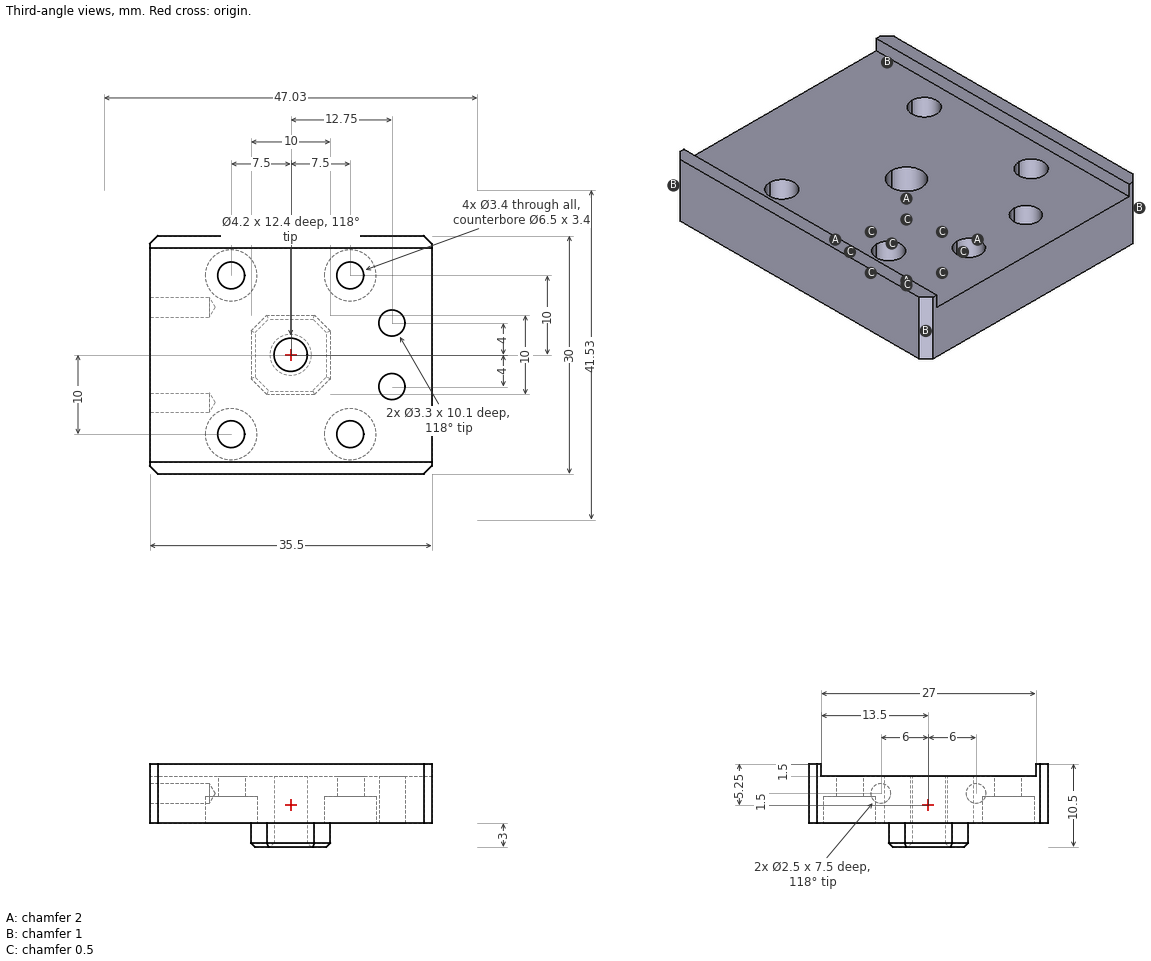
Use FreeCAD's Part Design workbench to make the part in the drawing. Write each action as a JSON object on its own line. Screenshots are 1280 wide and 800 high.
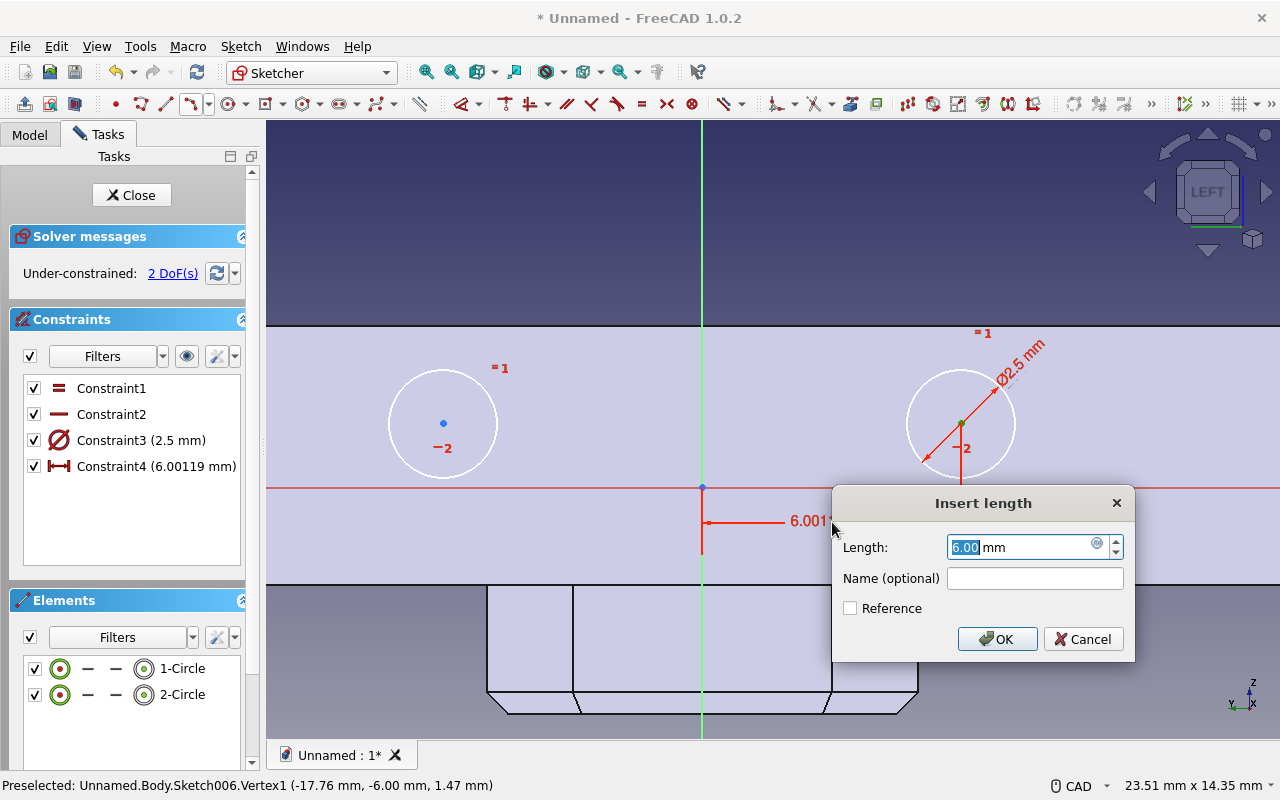
{"action": "type", "text": "6"}
{"action": "key", "text": "Return"}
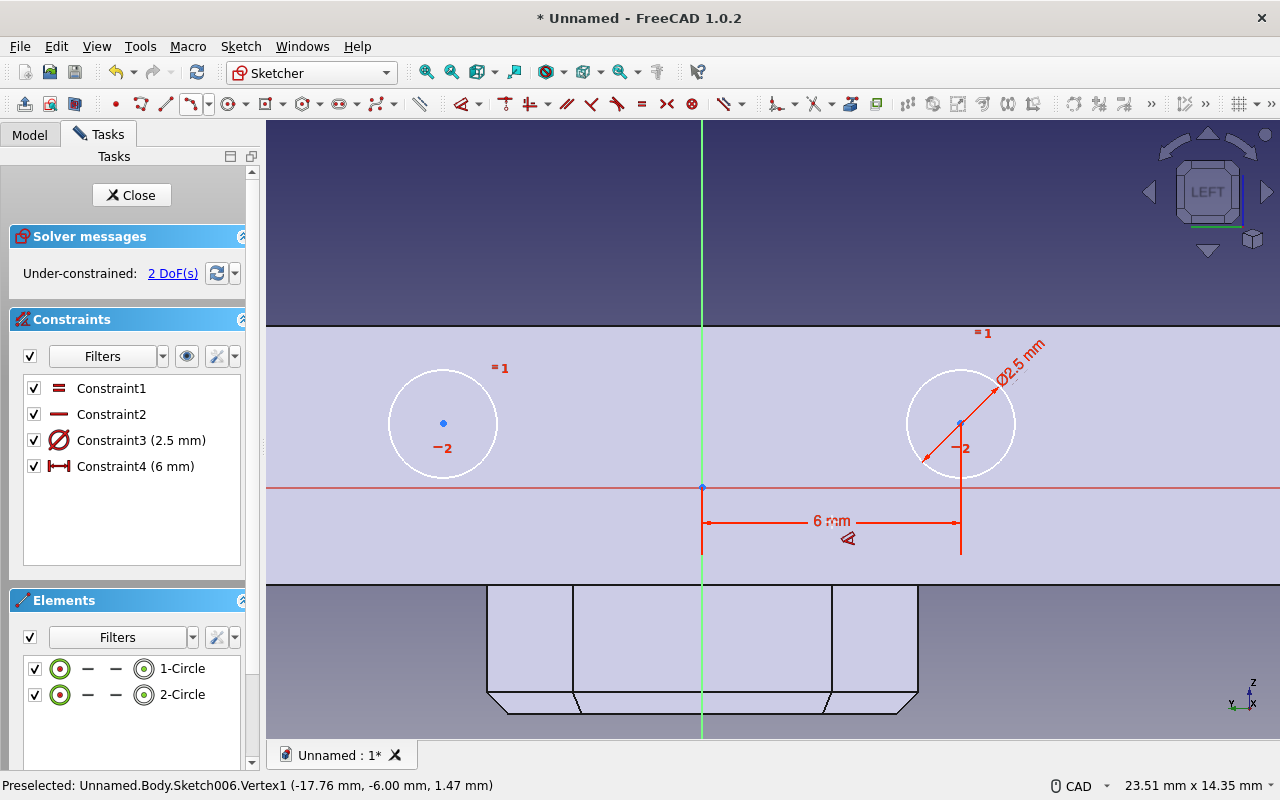
{"action": "left_click", "coordinate": [443, 424]}
{"action": "left_click", "coordinate": [573, 522]}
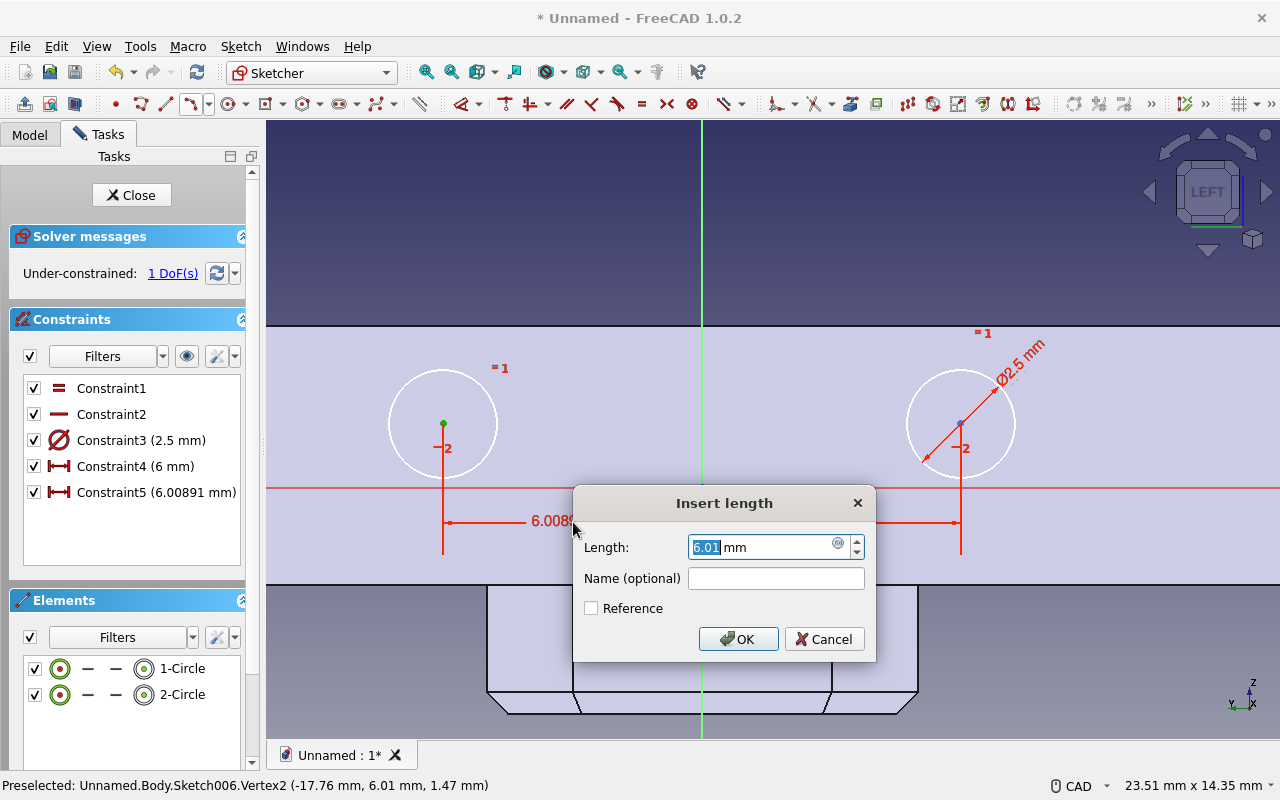
{"action": "type", "text": "6"}
{"action": "key", "text": "Return"}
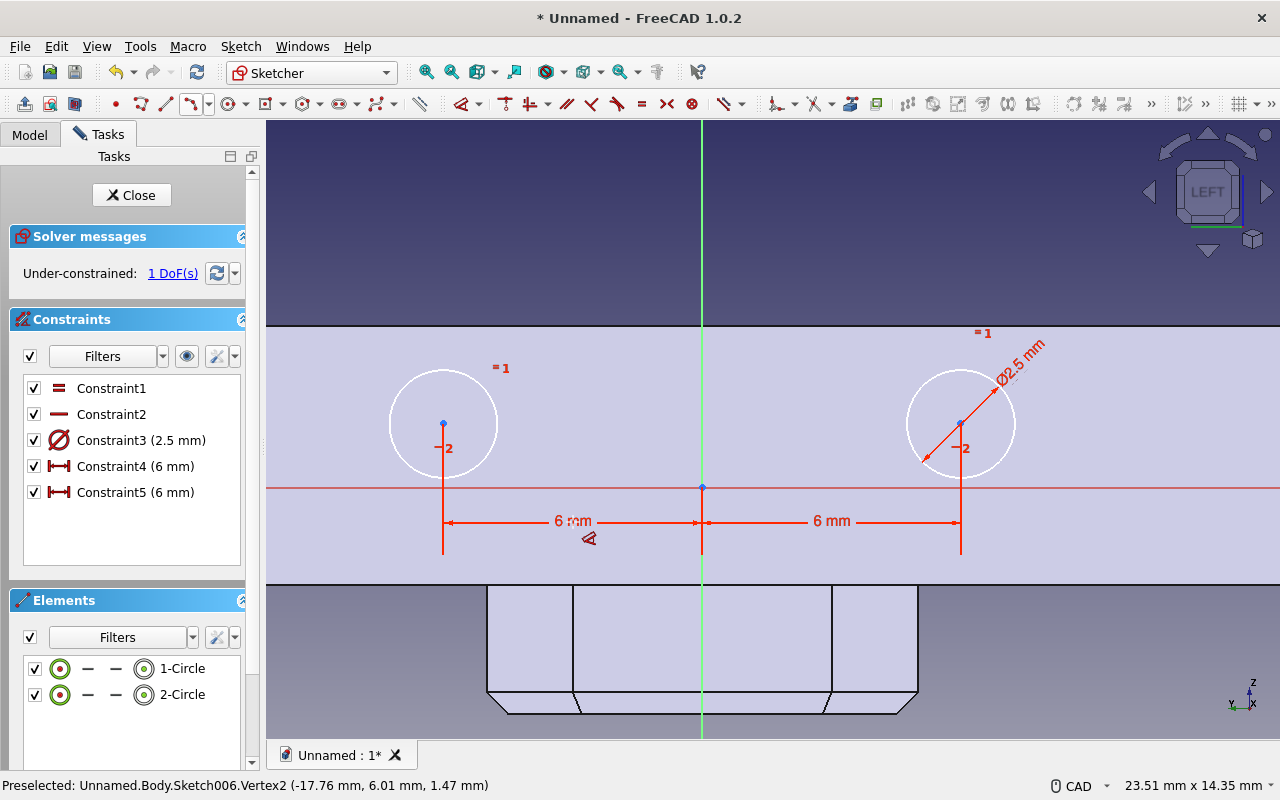
{"action": "left_click", "coordinate": [961, 424]}
{"action": "left_click", "coordinate": [995, 441]}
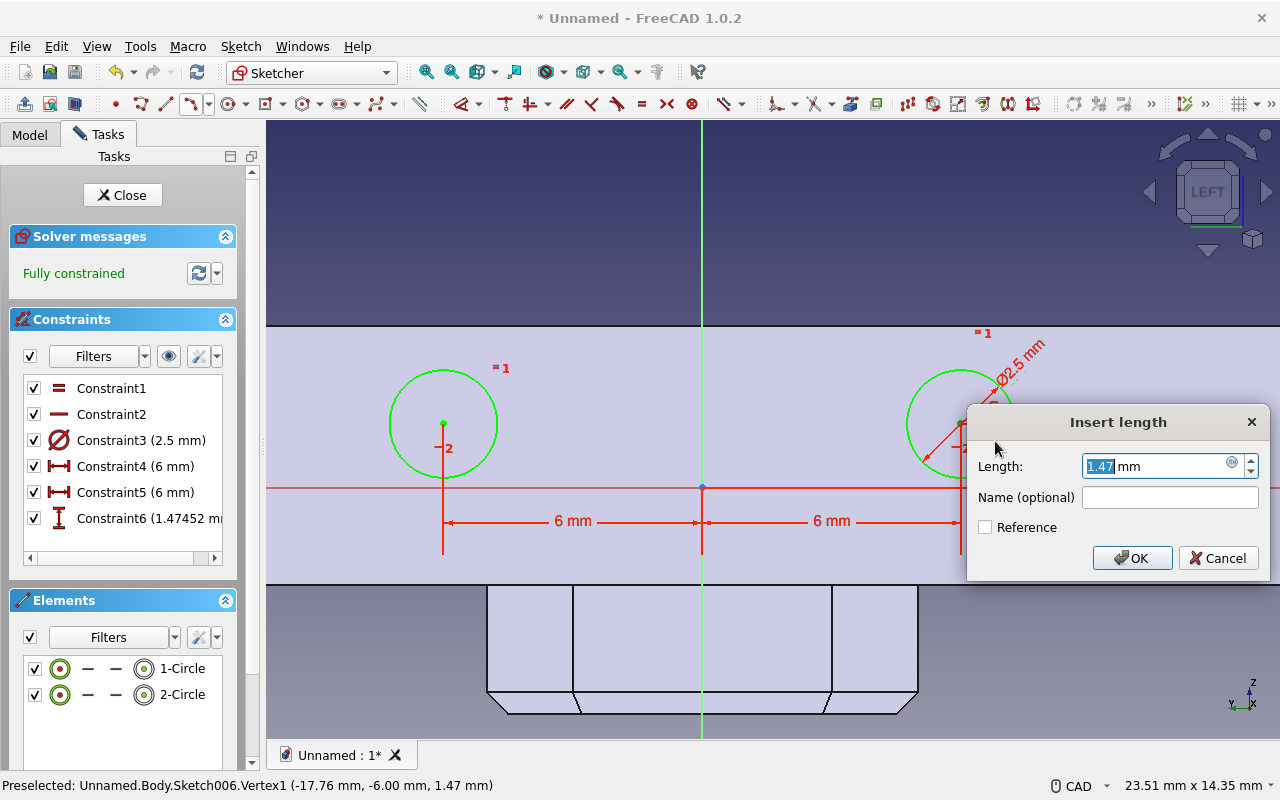
{"action": "type", "text": "1.5"}
{"action": "key", "text": "Return"}
{"action": "key", "text": "Escape"}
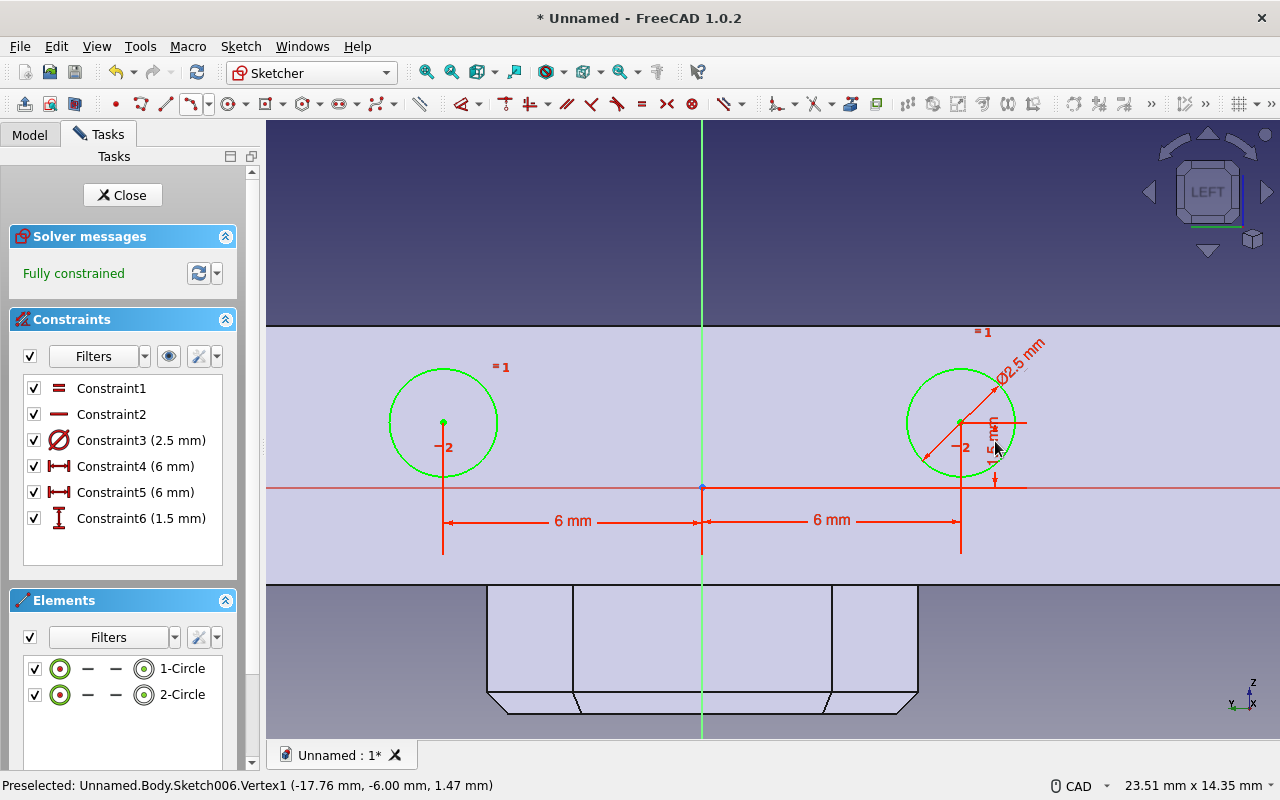
{"action": "left_click", "coordinate": [123, 195]}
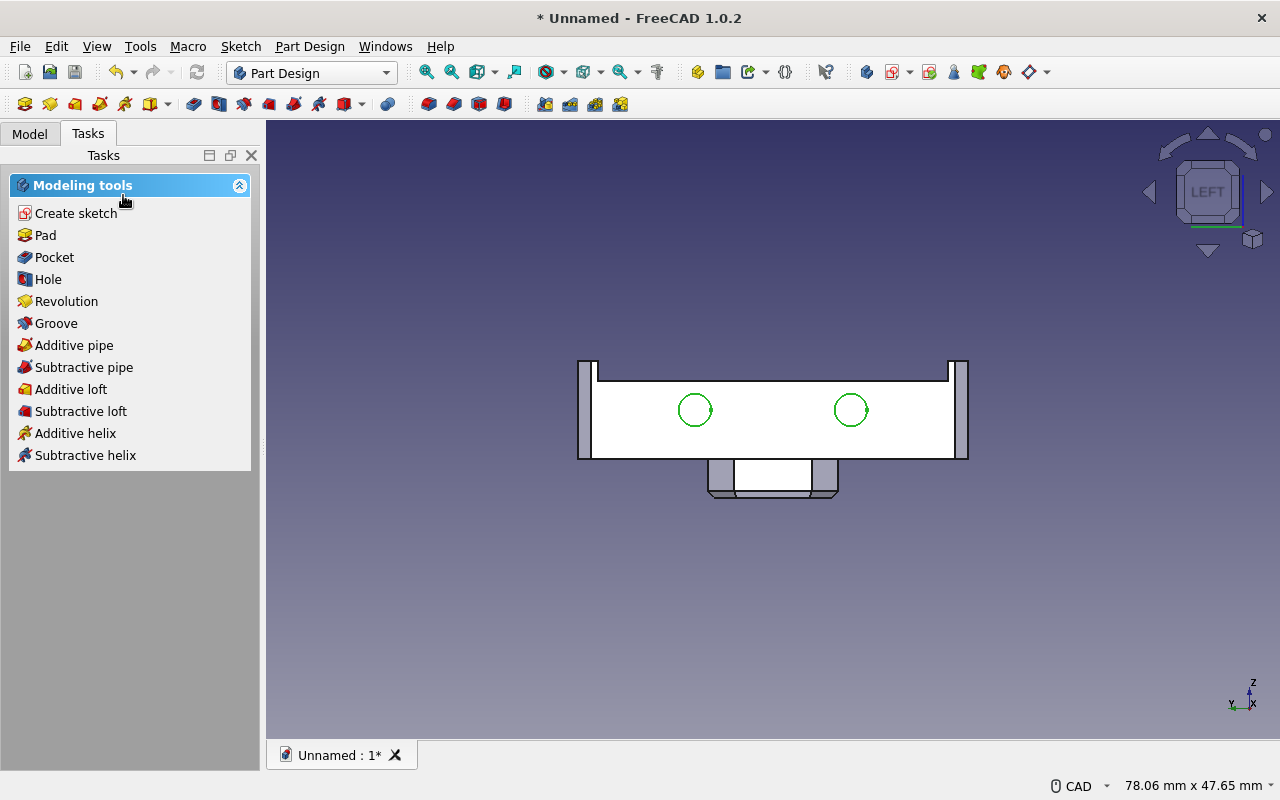
{"action": "left_click", "coordinate": [219, 104]}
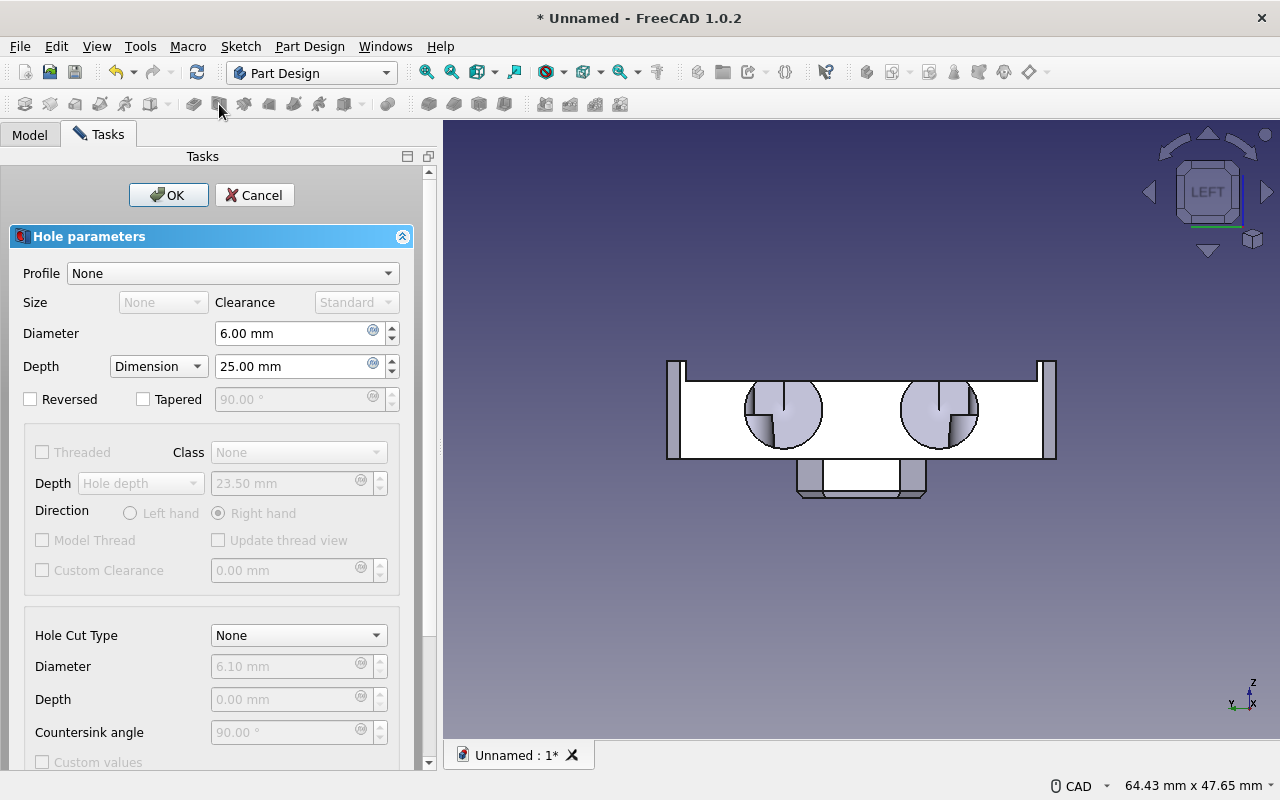
{"action": "triple_click", "coordinate": [300, 334]}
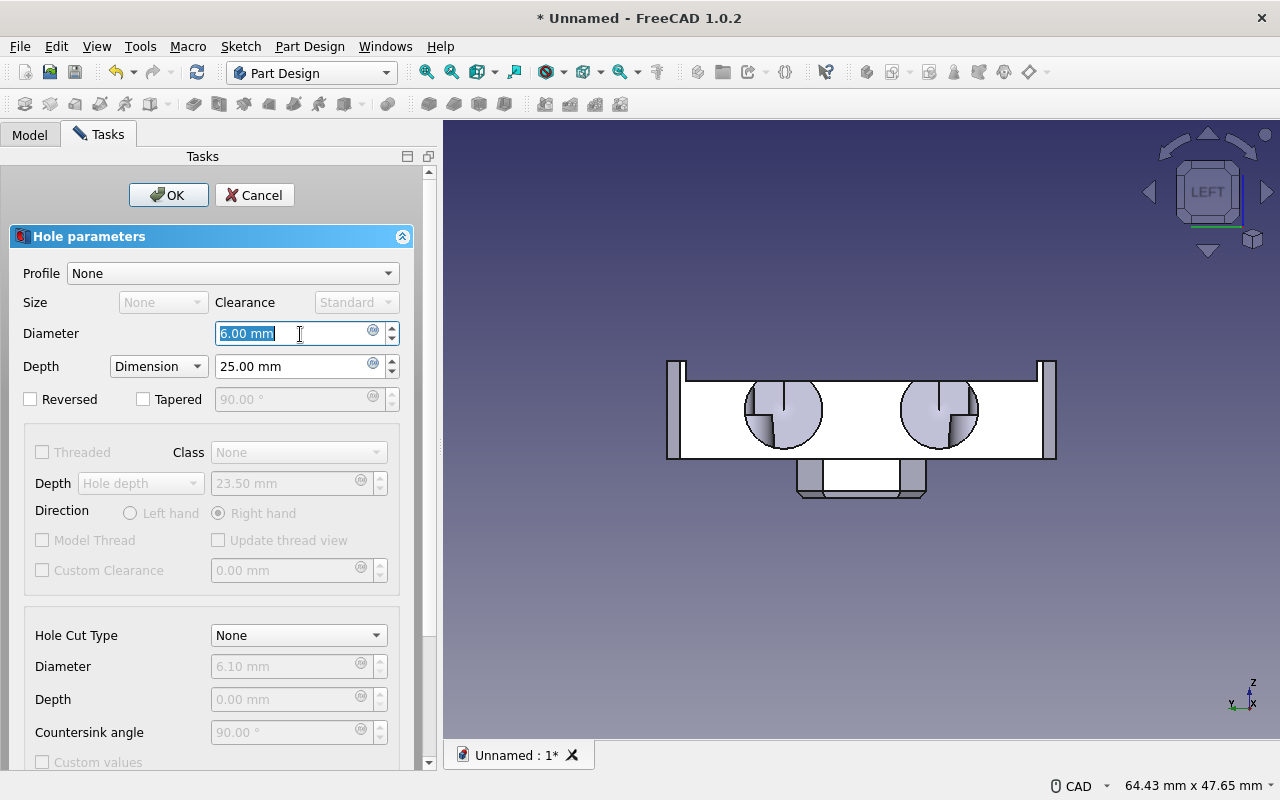
{"action": "type", "text": "2.5"}
{"action": "key", "text": "Tab"}